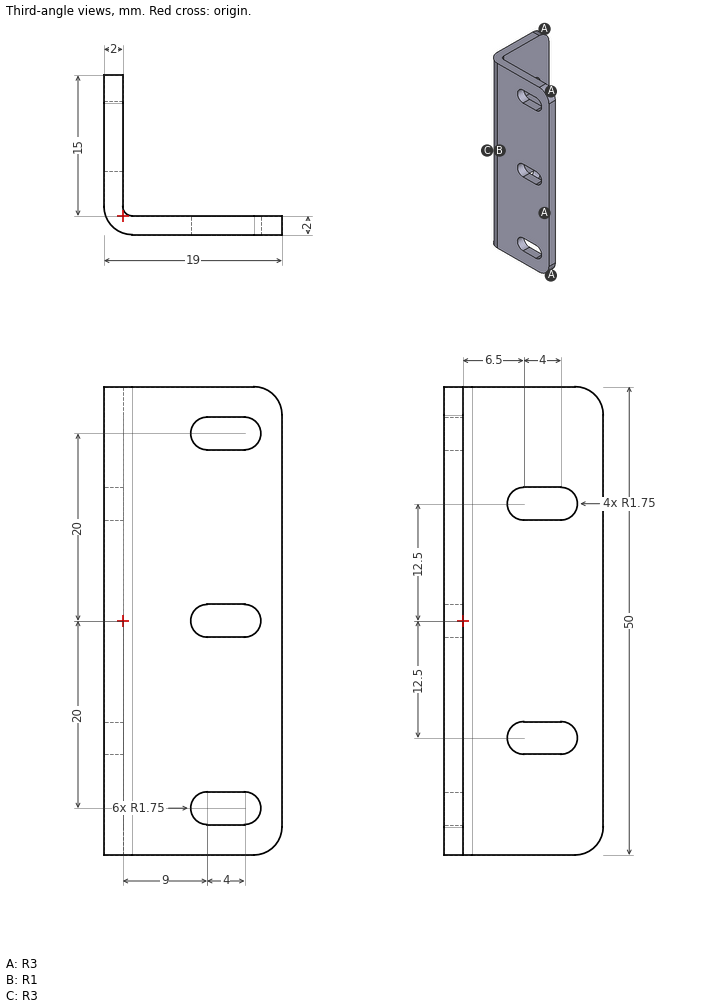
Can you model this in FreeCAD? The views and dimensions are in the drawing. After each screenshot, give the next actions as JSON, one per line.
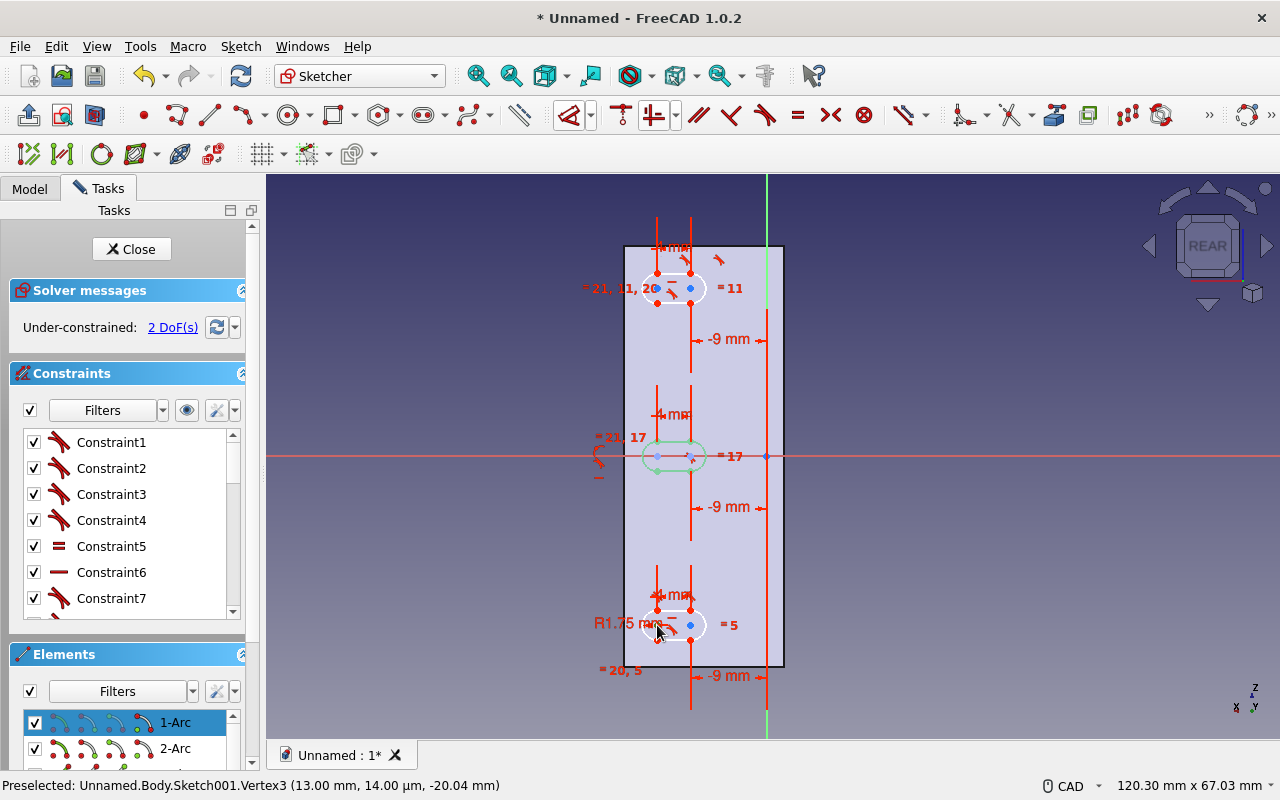
{"action": "left_click", "coordinate": [590, 116]}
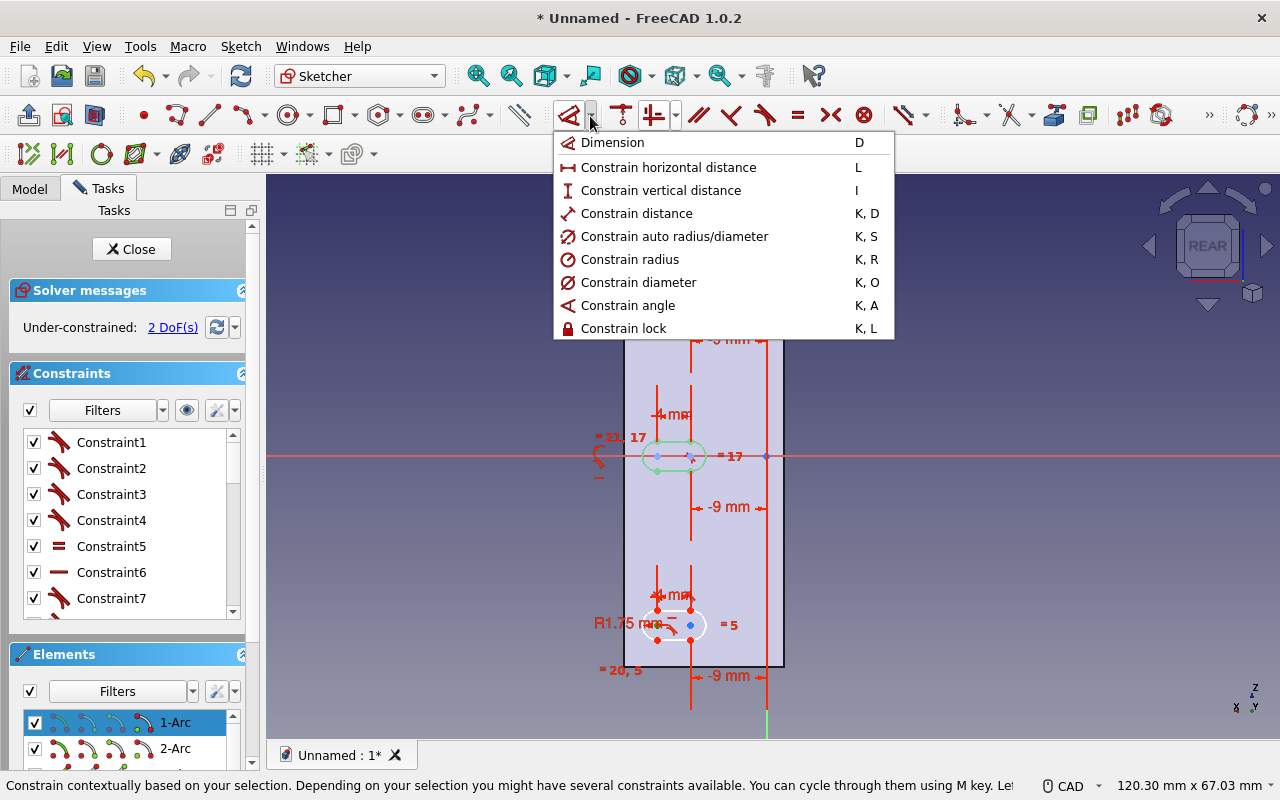
{"action": "left_click", "coordinate": [724, 190]}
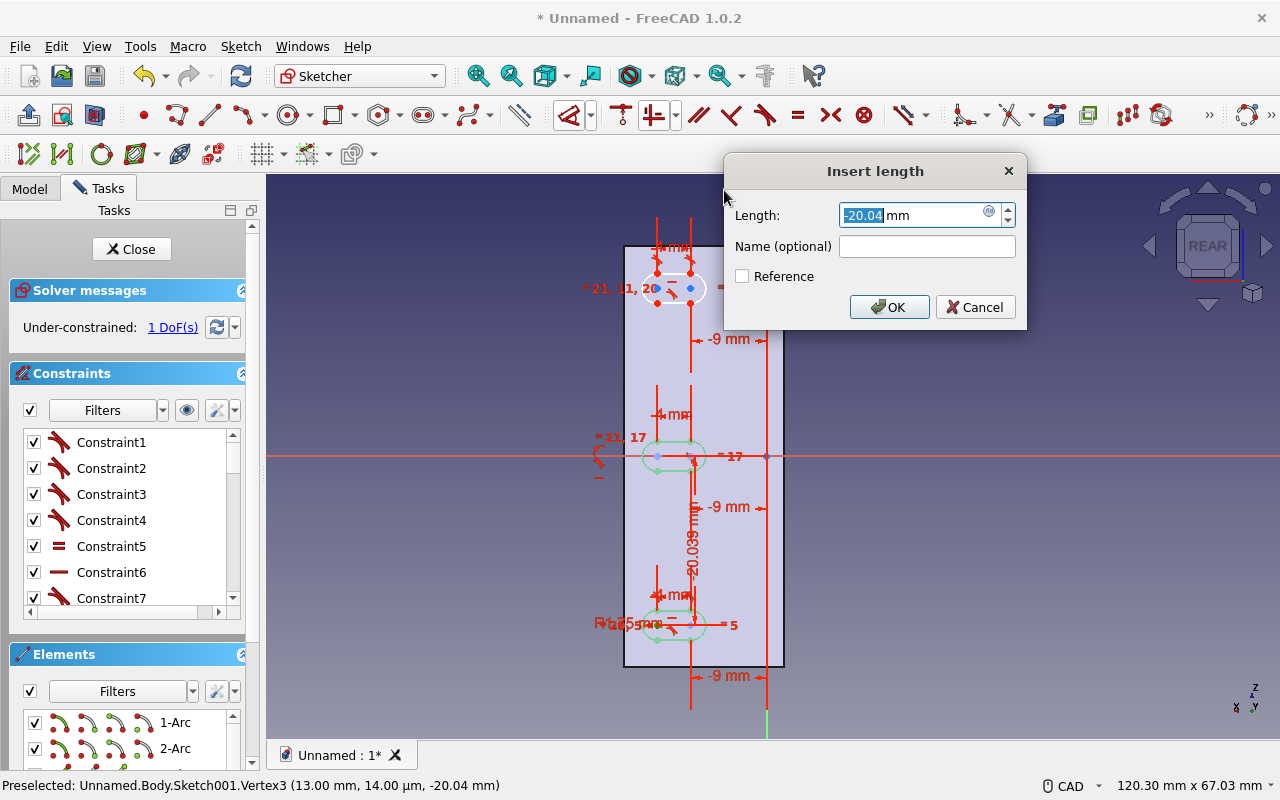
{"action": "type", "text": "-20"}
{"action": "key", "text": "Return"}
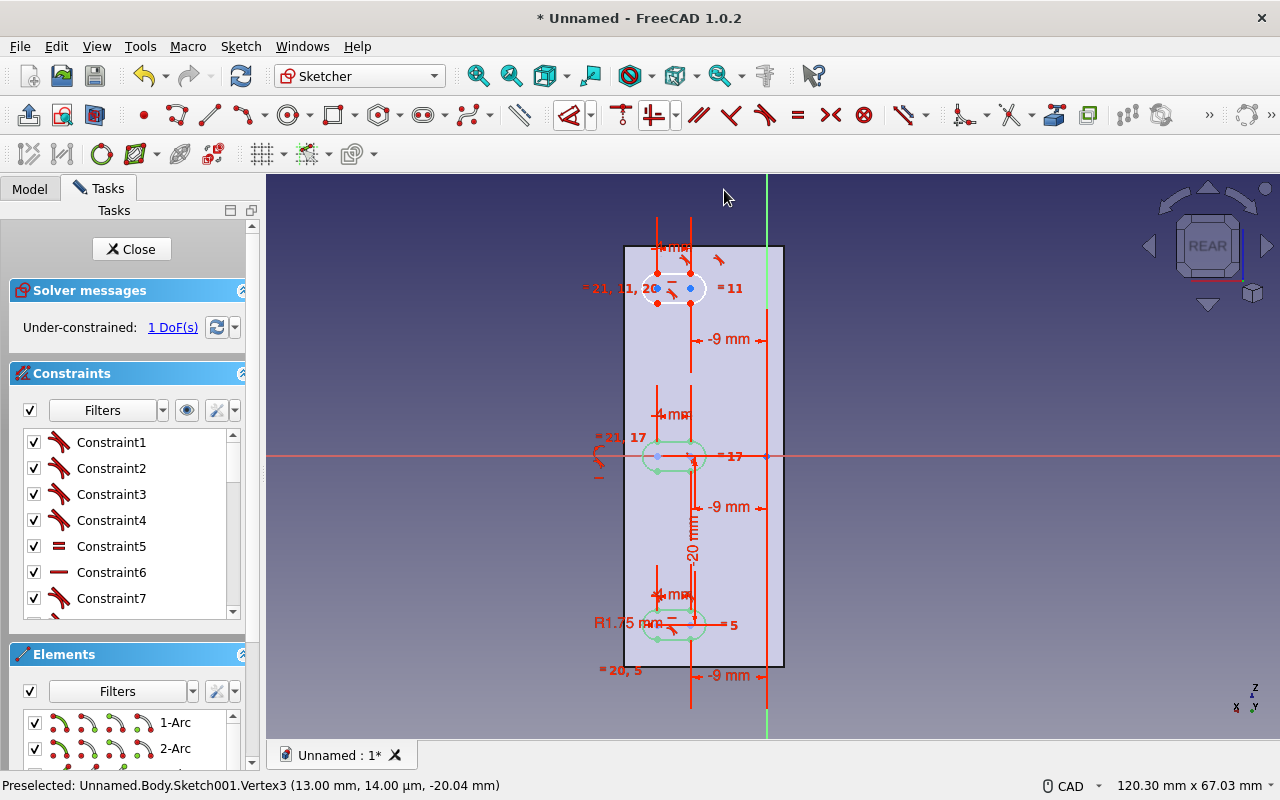
{"action": "left_click", "coordinate": [657, 289]}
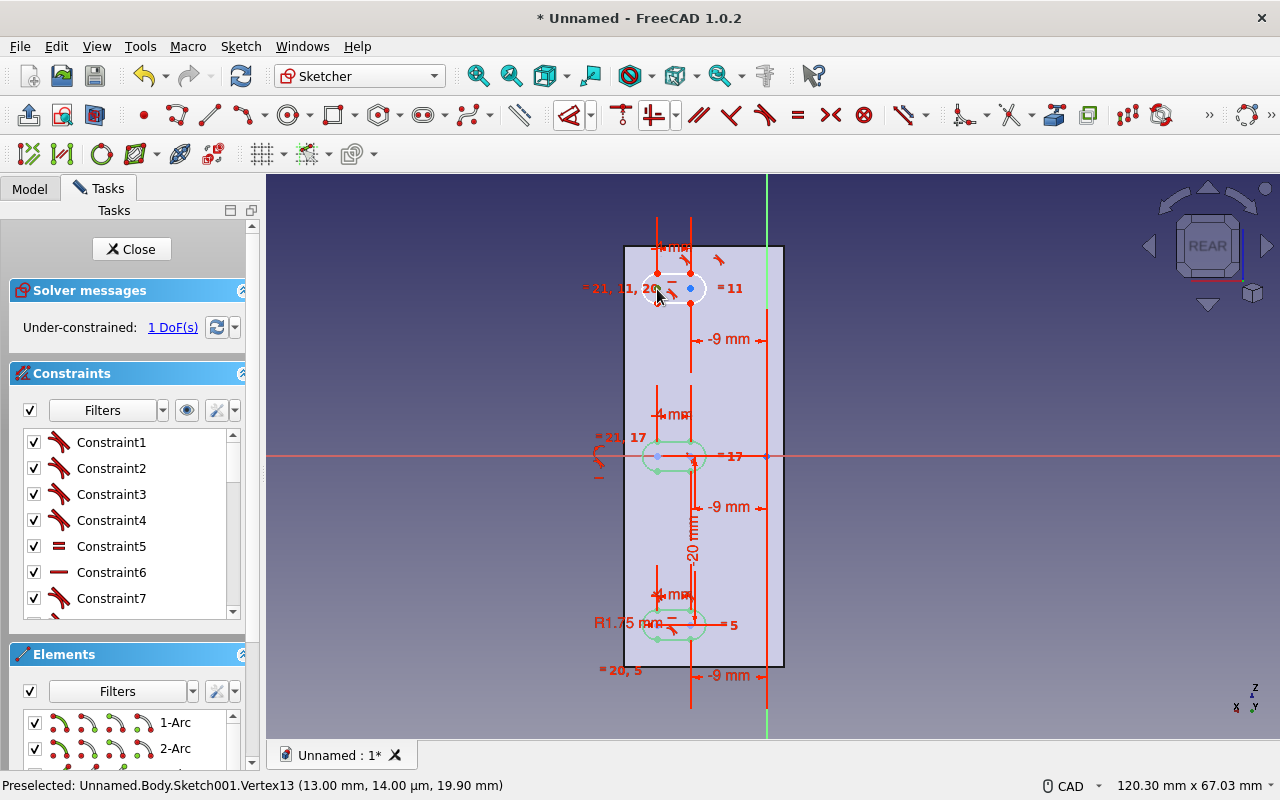
{"action": "key", "text": "i"}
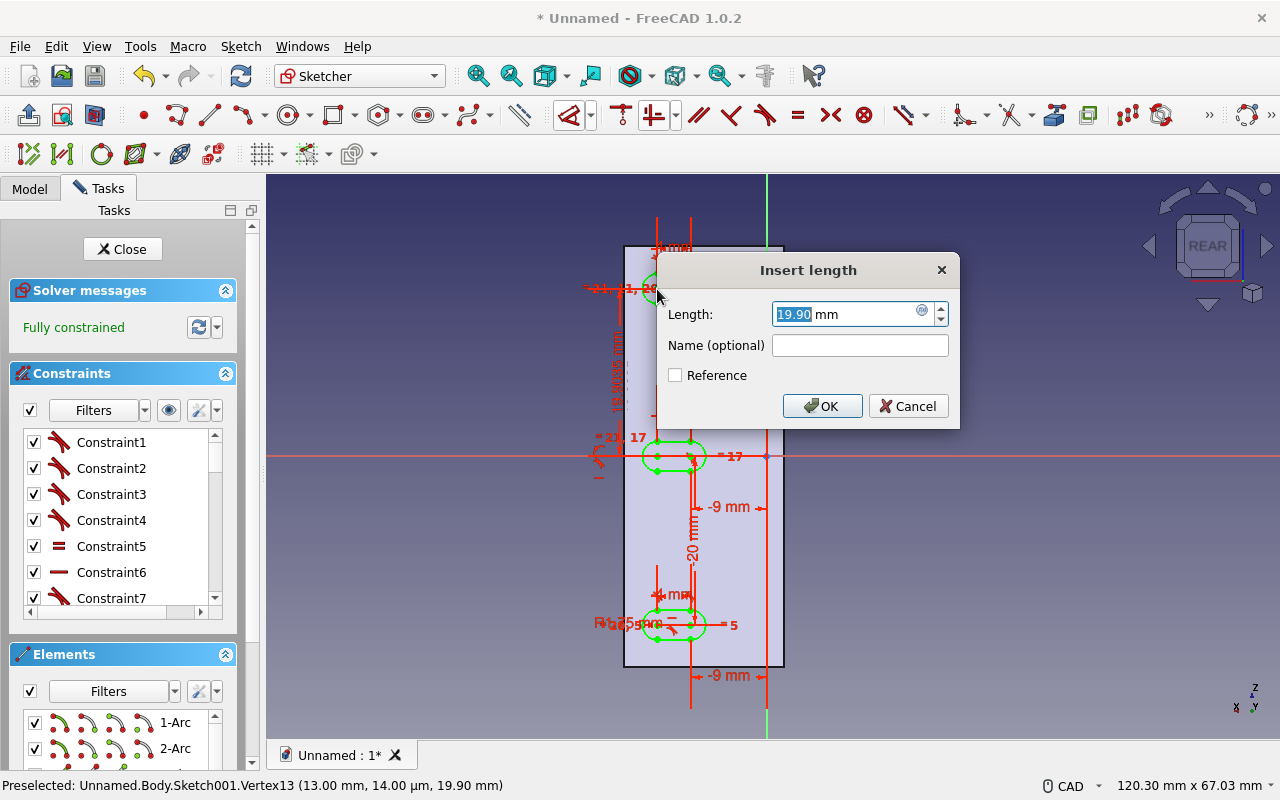
{"action": "type", "text": "20"}
{"action": "key", "text": "Return"}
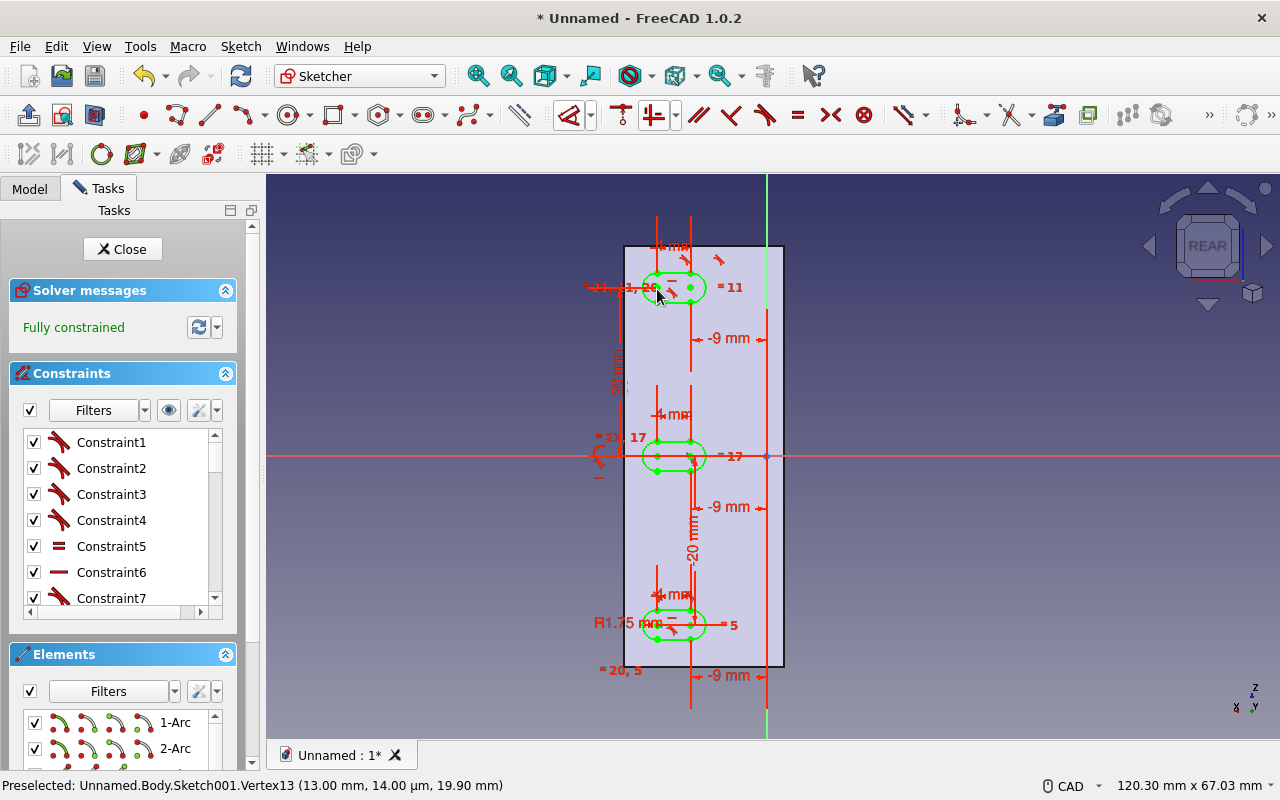
{"action": "left_click", "coordinate": [123, 249]}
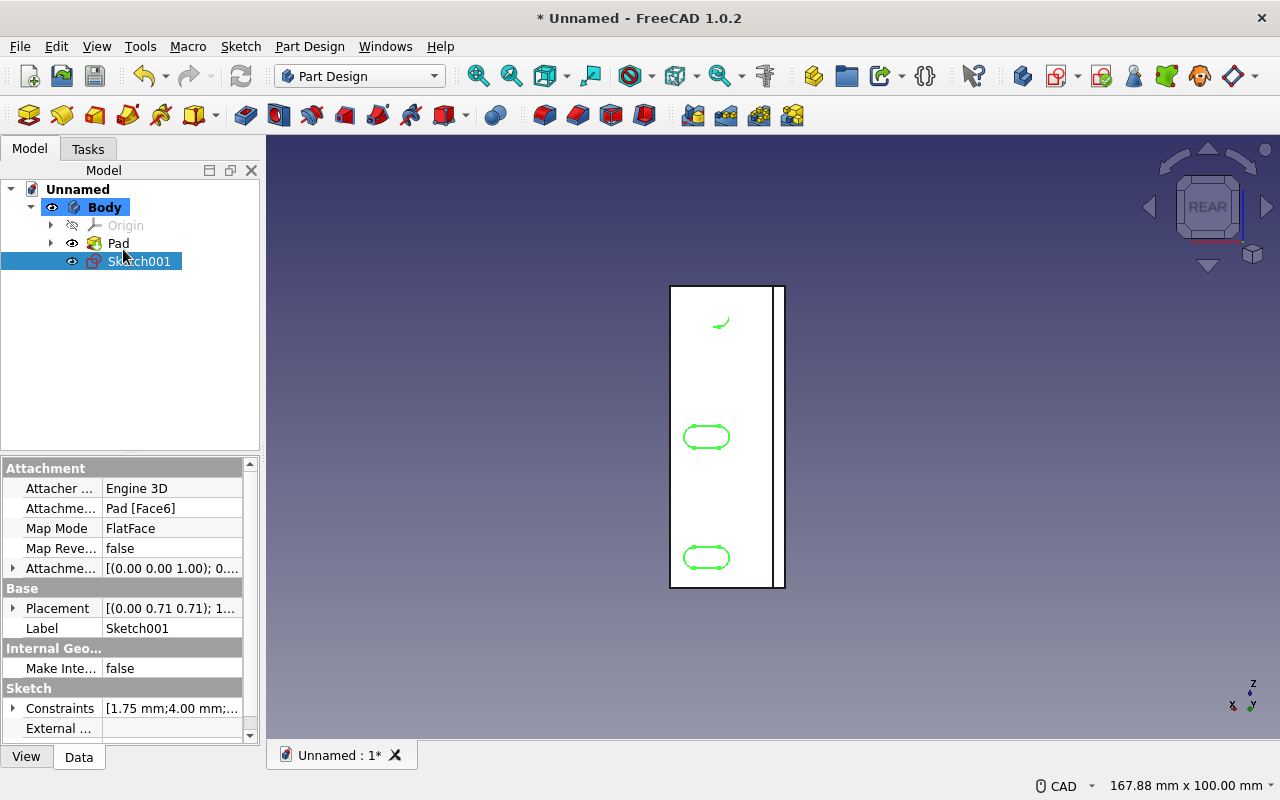
{"action": "left_click", "coordinate": [246, 116]}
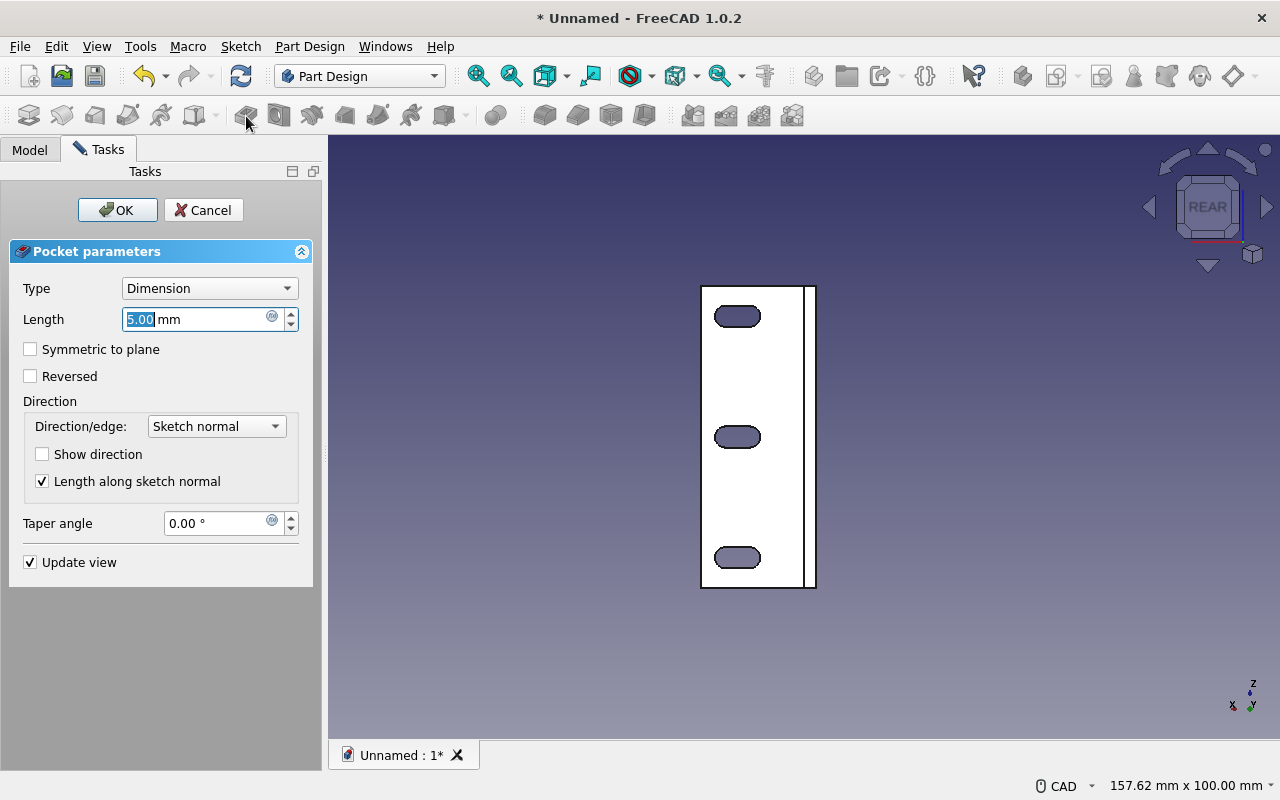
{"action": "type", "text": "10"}
{"action": "key", "text": "Tab"}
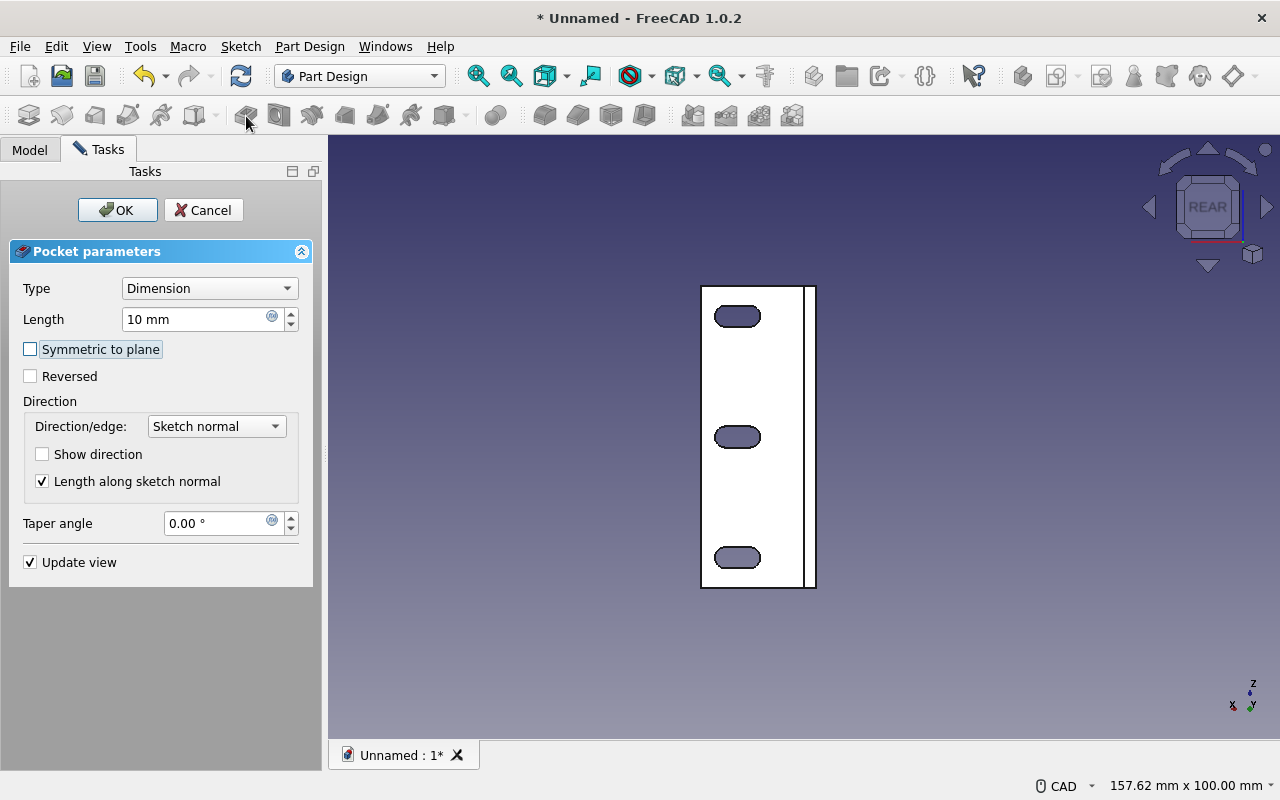
{"action": "left_click", "coordinate": [118, 210]}